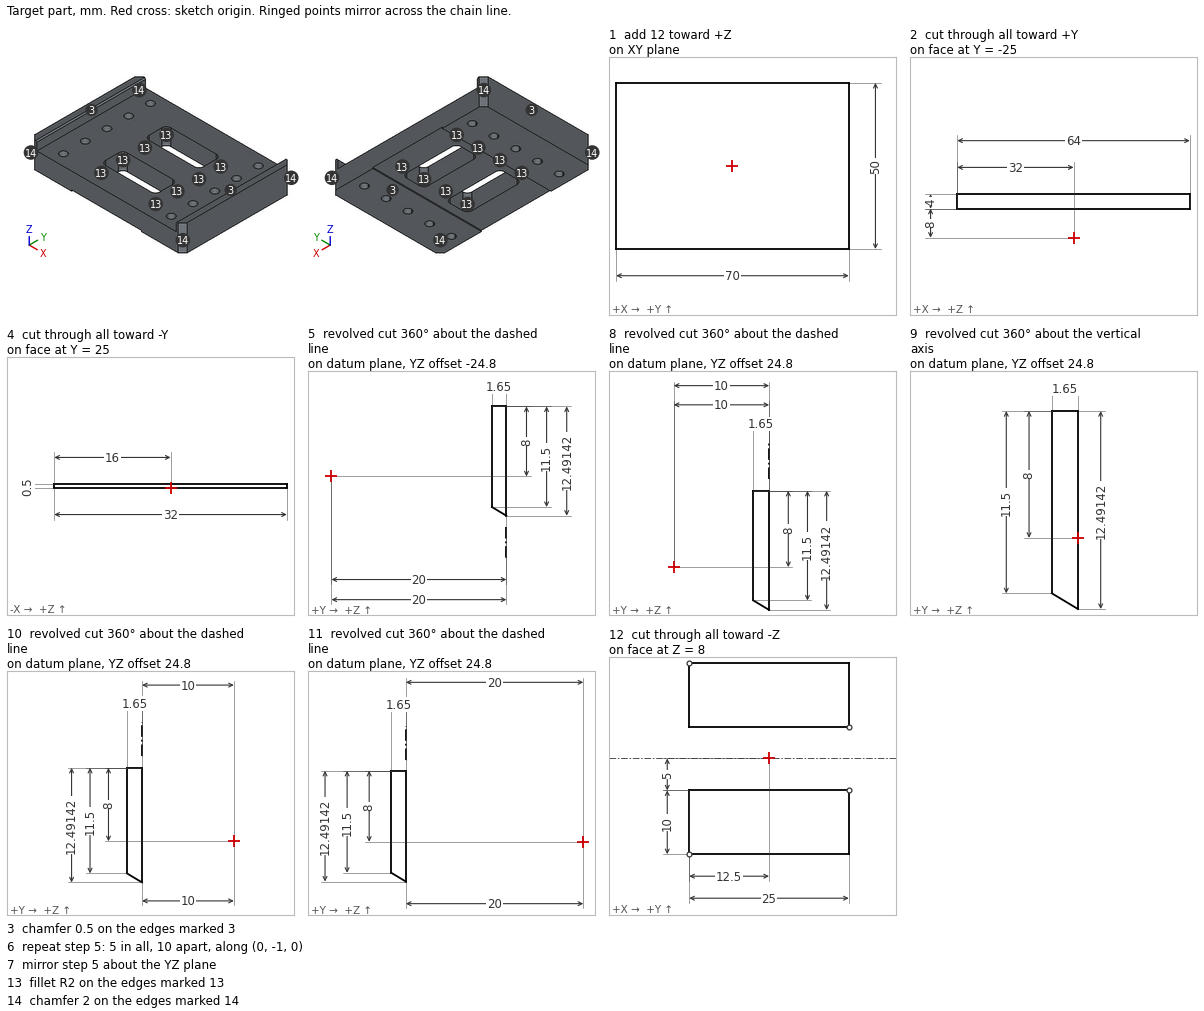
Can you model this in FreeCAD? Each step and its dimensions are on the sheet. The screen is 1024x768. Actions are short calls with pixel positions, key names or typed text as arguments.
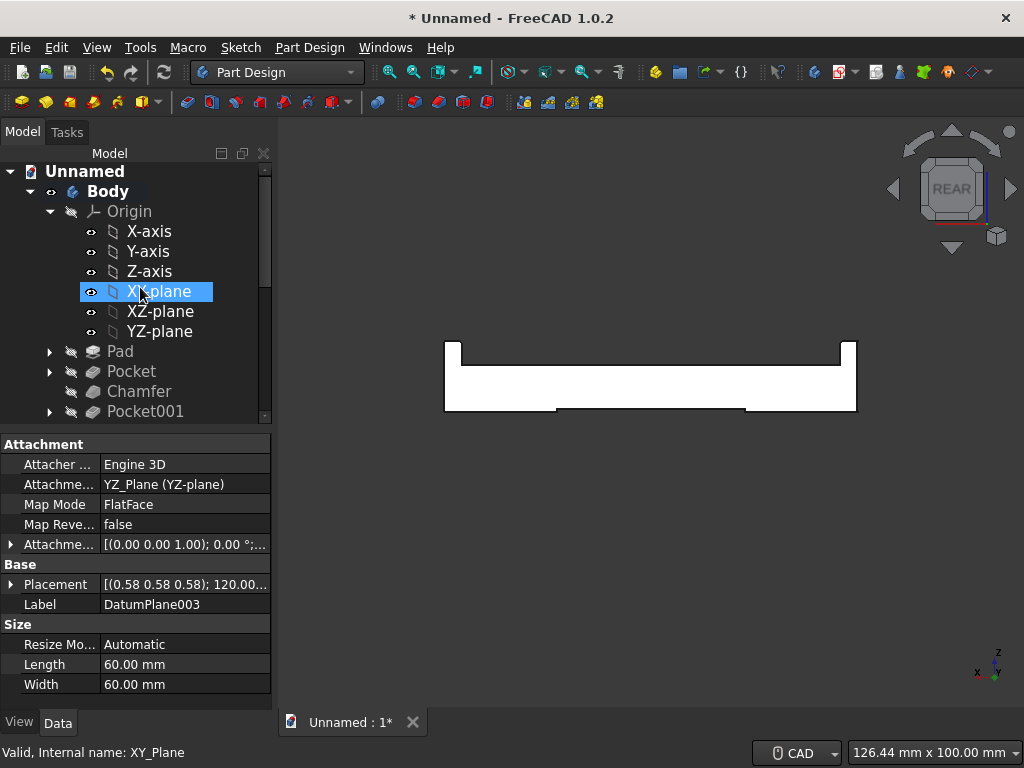
click(136, 332)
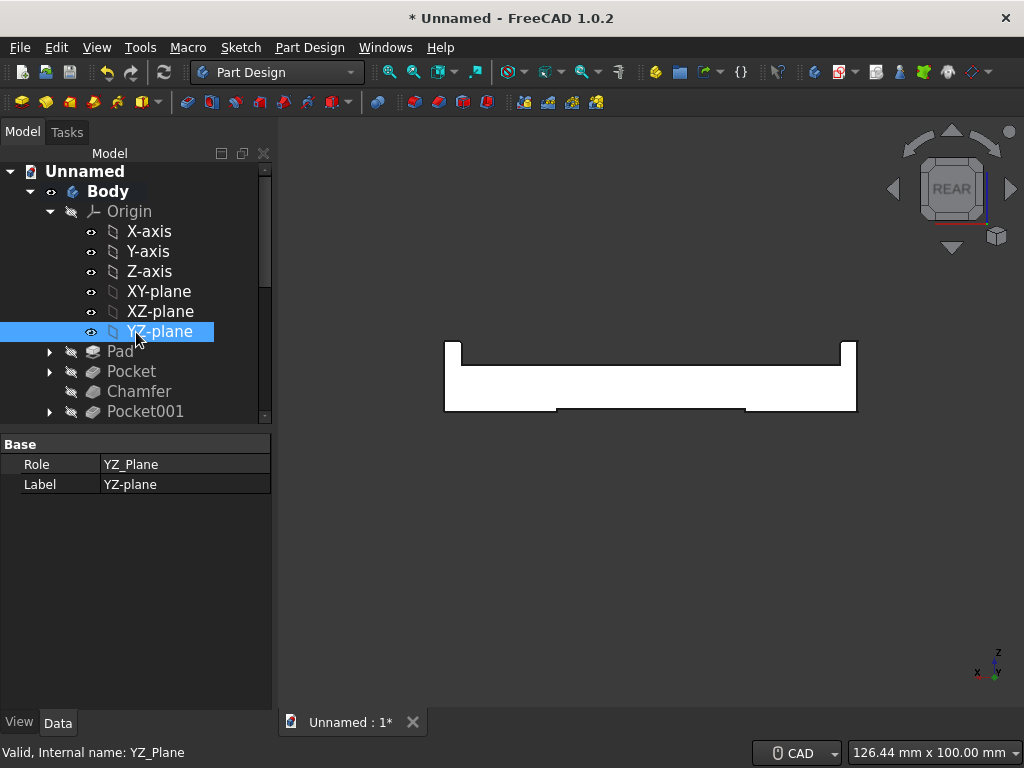
click(972, 72)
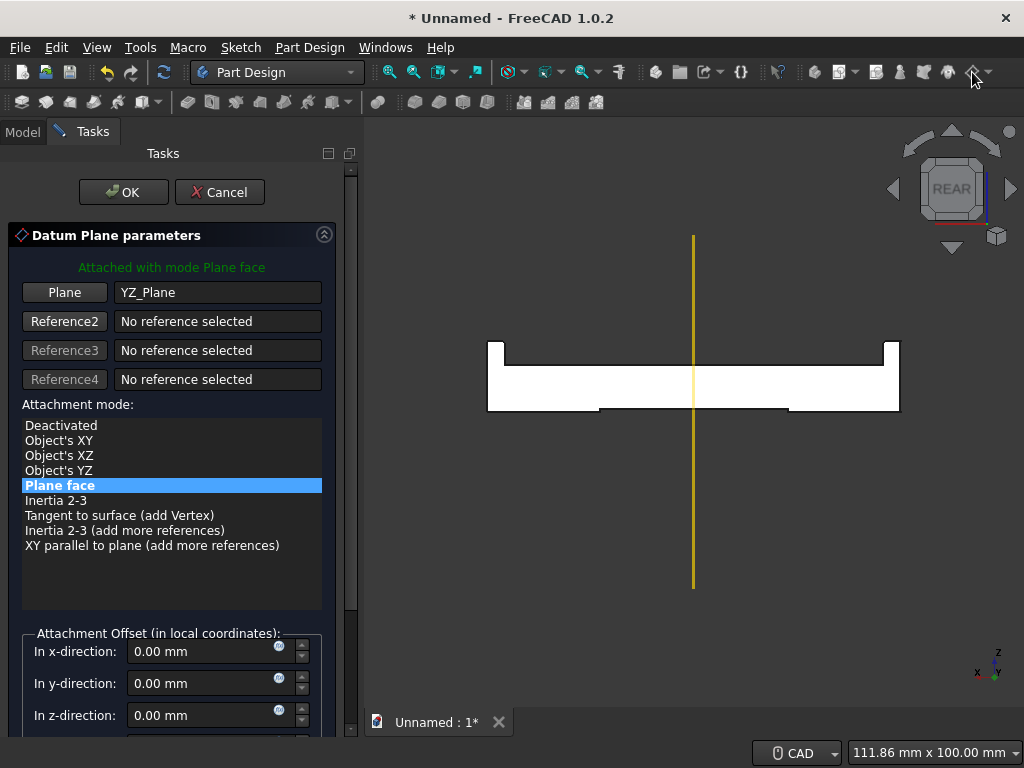
triple_click(210, 715)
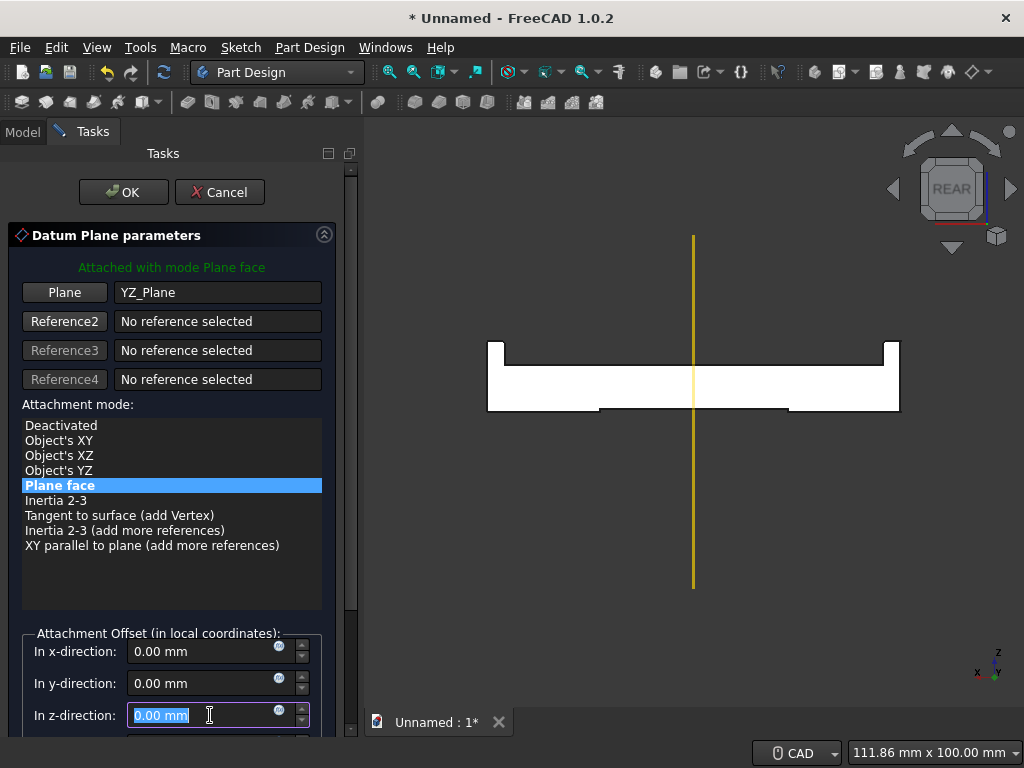
text(24.8)
key(Tab)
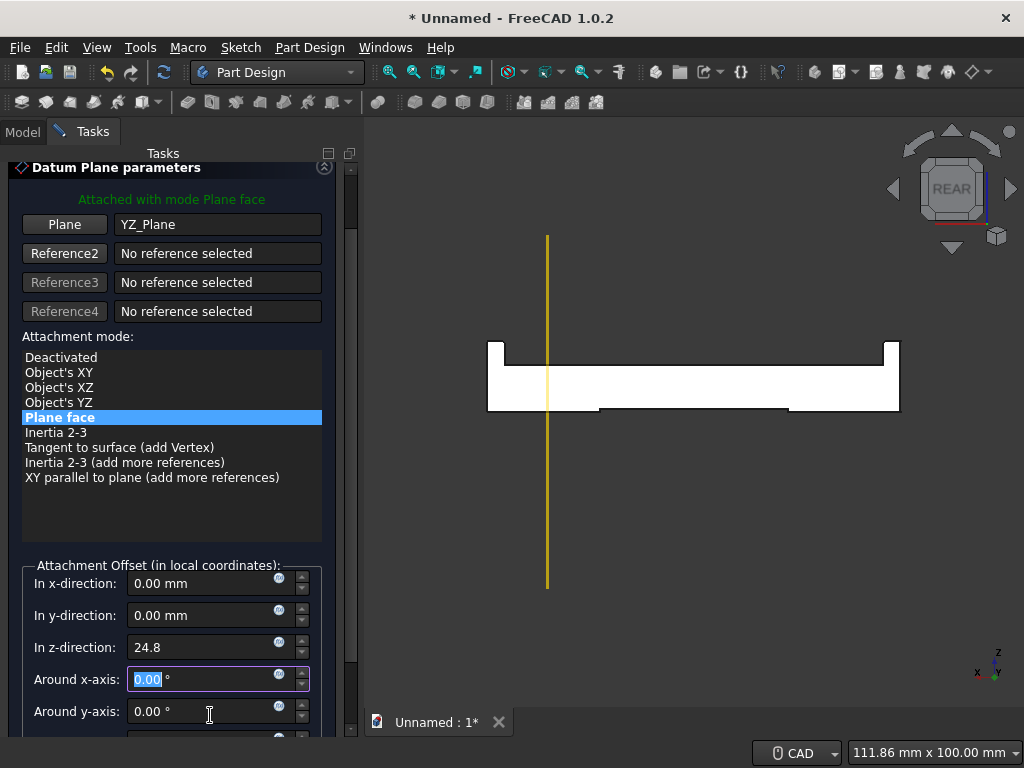
scroll(351, 450, up, 2)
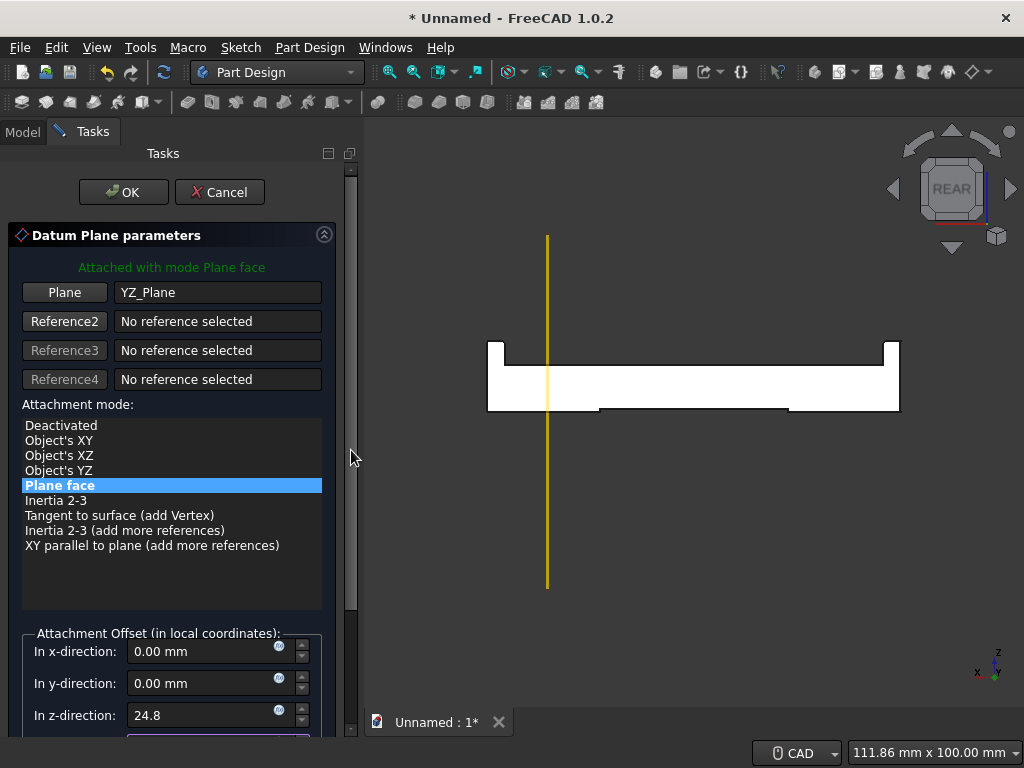
click(124, 192)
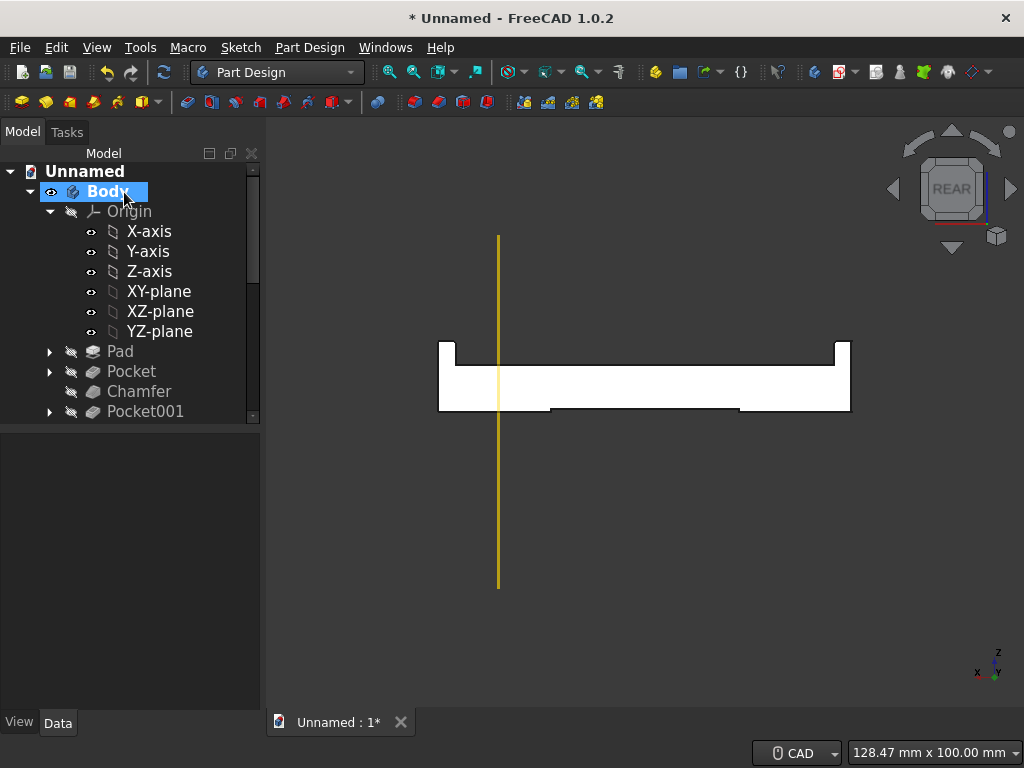
scroll(100, 287, down, 3)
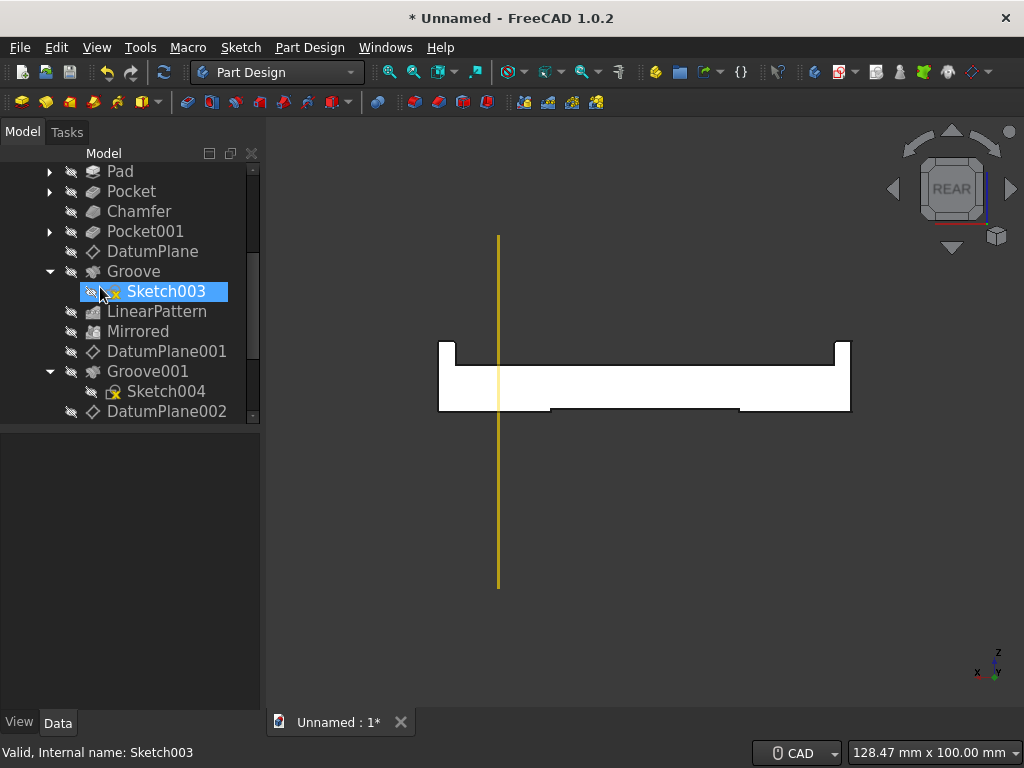
scroll(140, 287, up, 15)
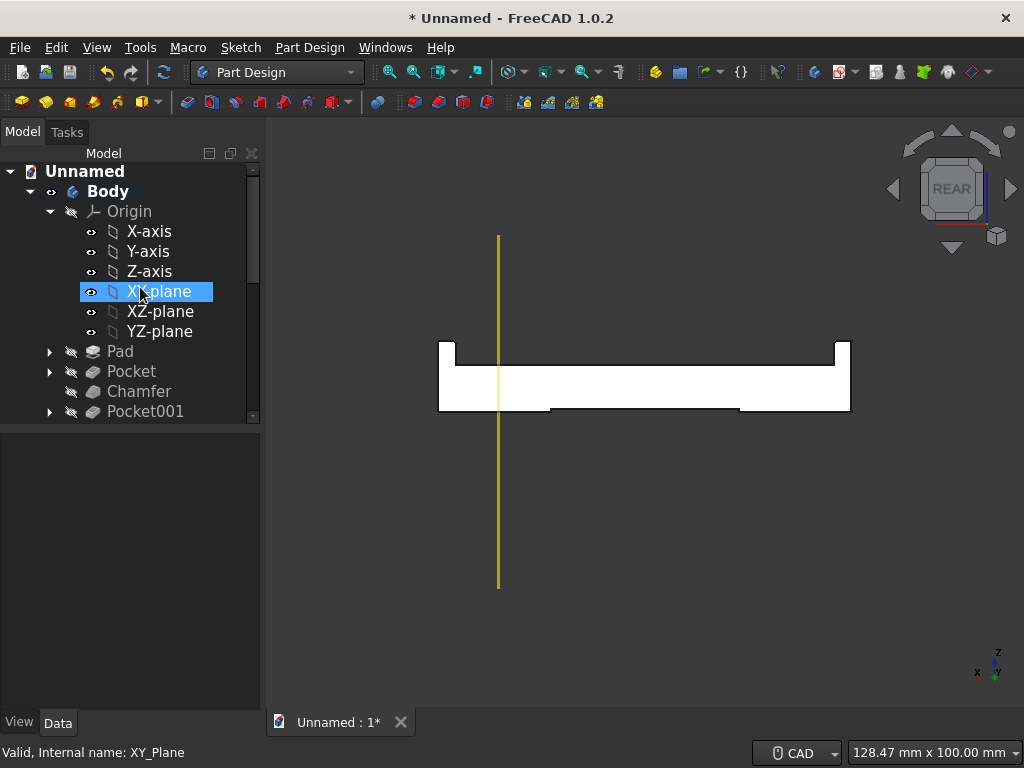
scroll(100, 287, down, 6)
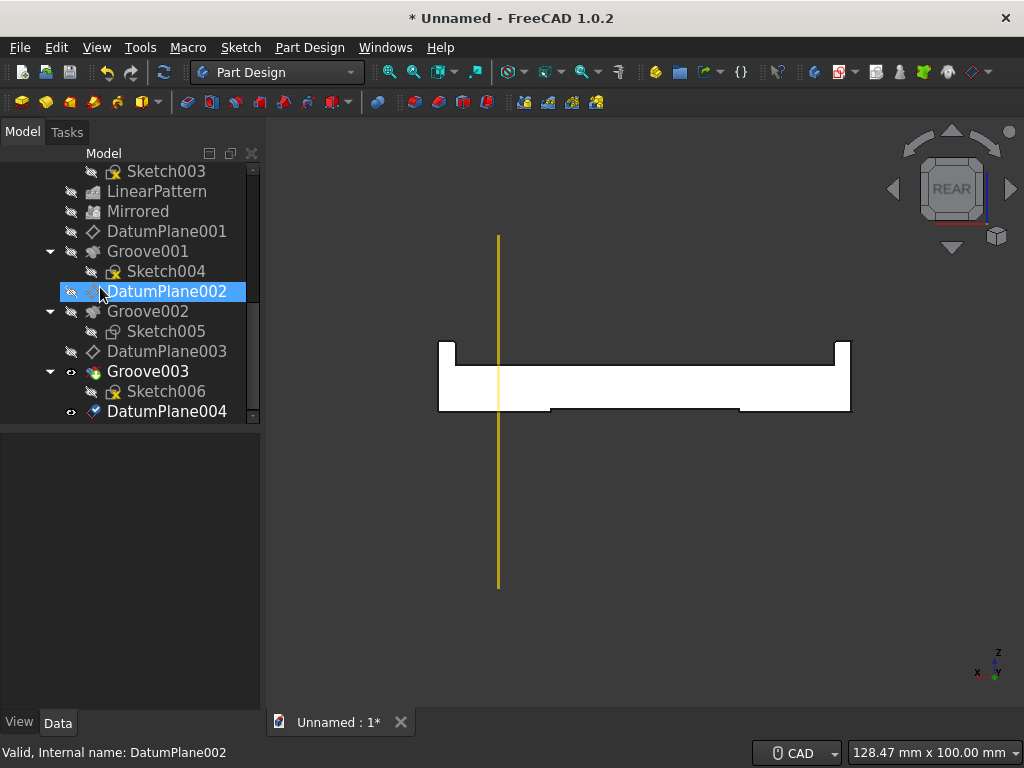
click(116, 412)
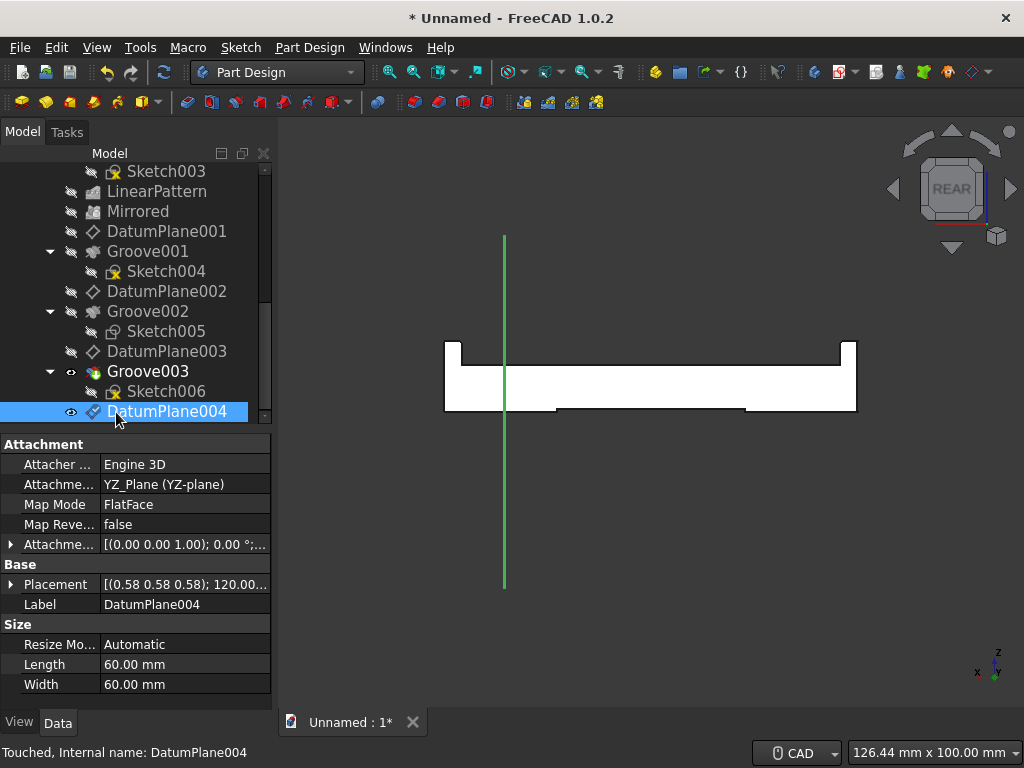
click(840, 72)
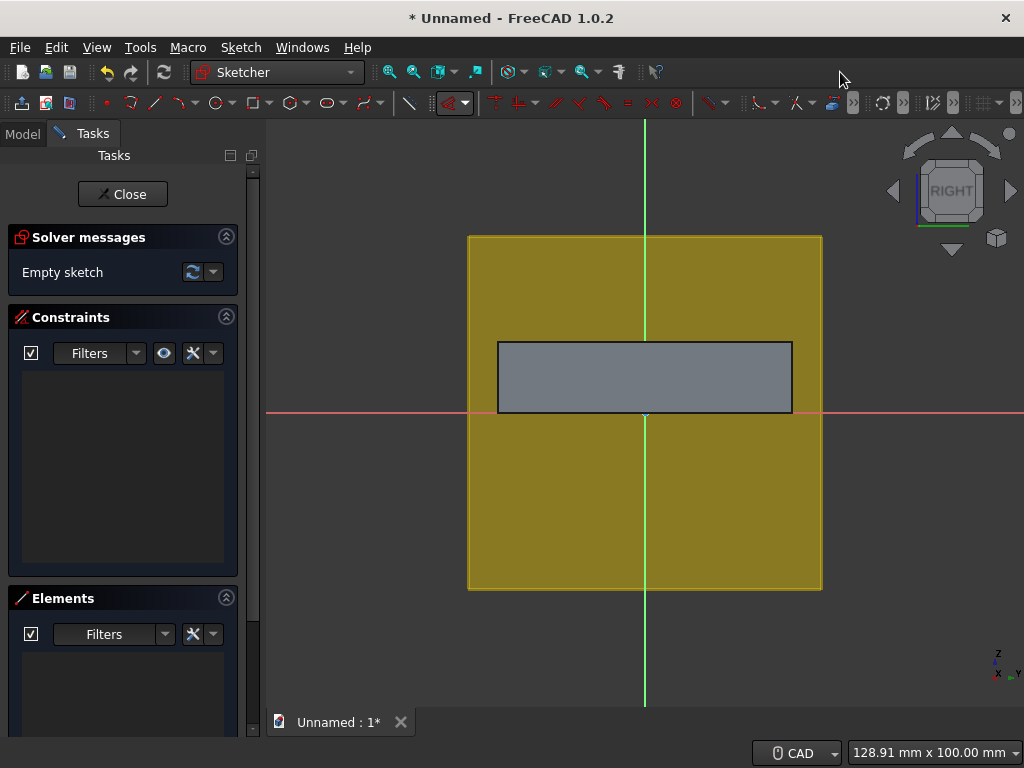
click(70, 104)